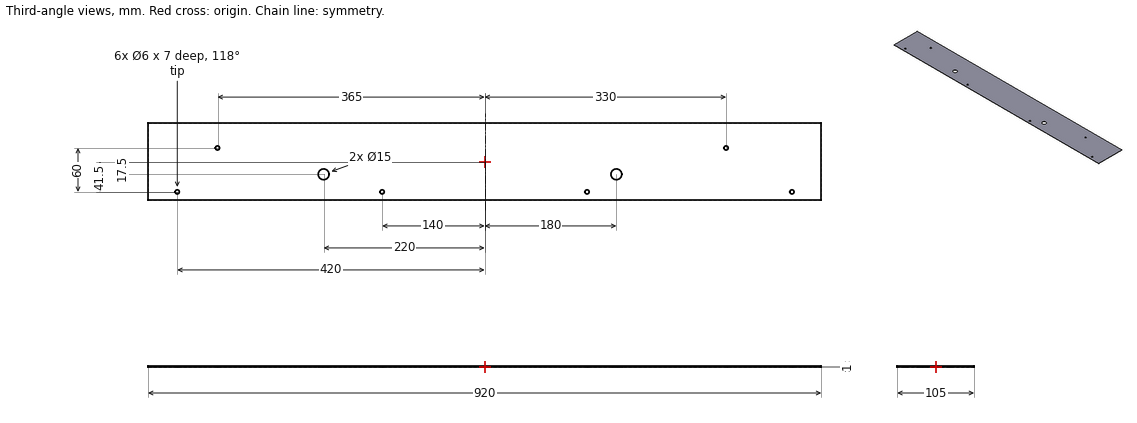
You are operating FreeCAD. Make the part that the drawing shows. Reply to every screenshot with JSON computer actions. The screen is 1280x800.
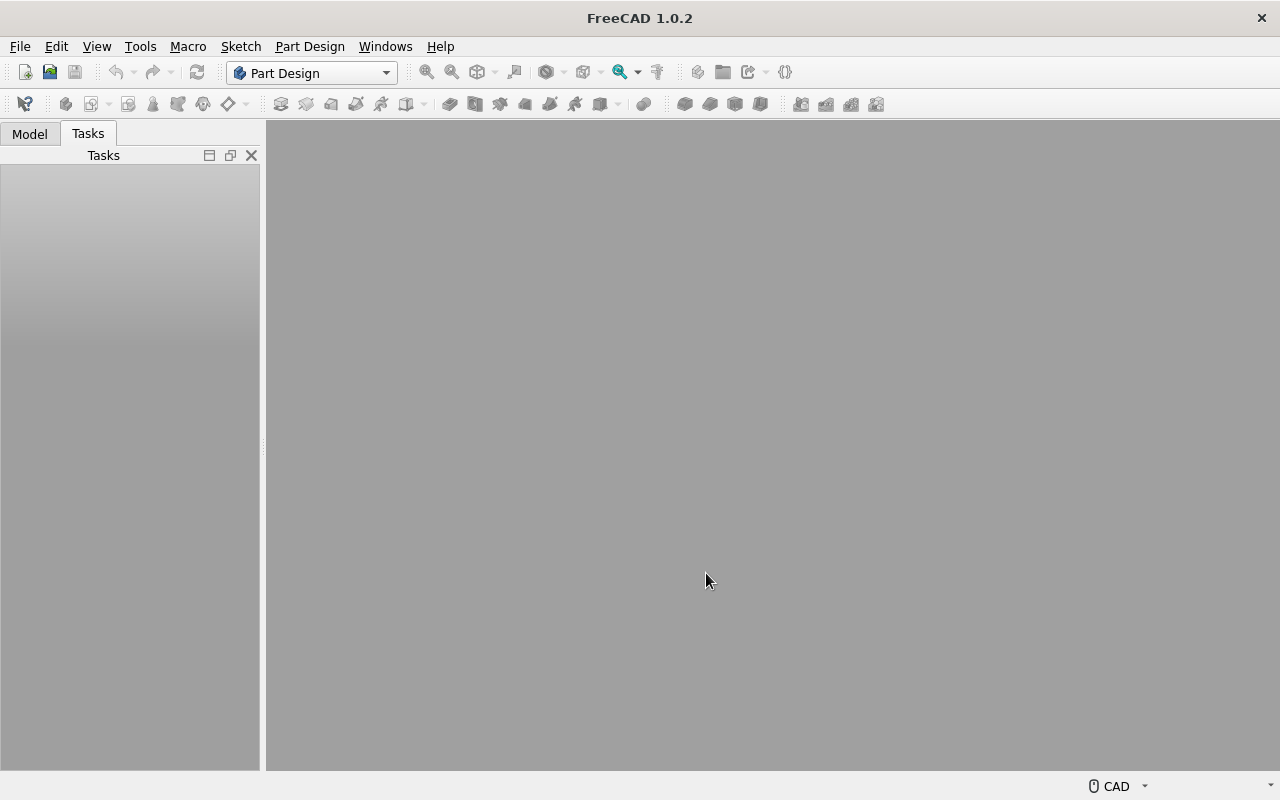
{"action": "left_click", "coordinate": [25, 72]}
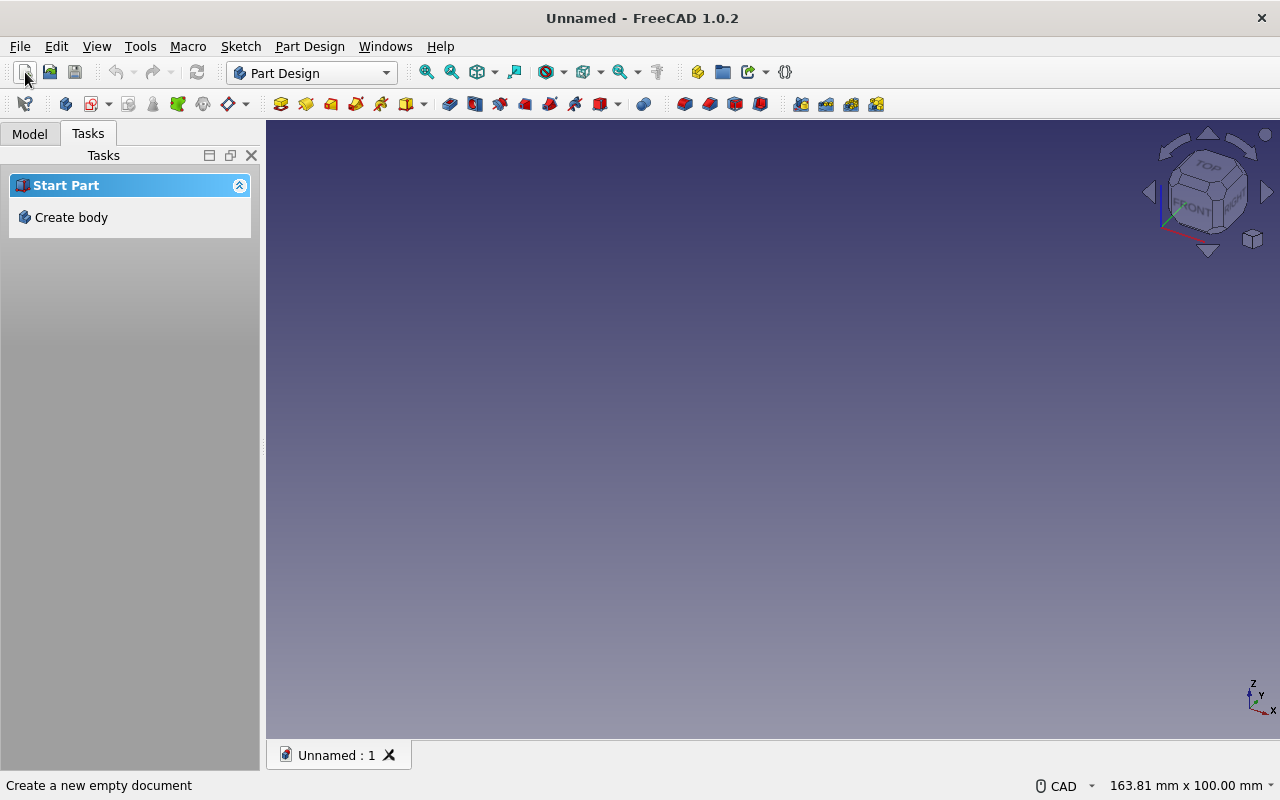
{"action": "left_click", "coordinate": [90, 104]}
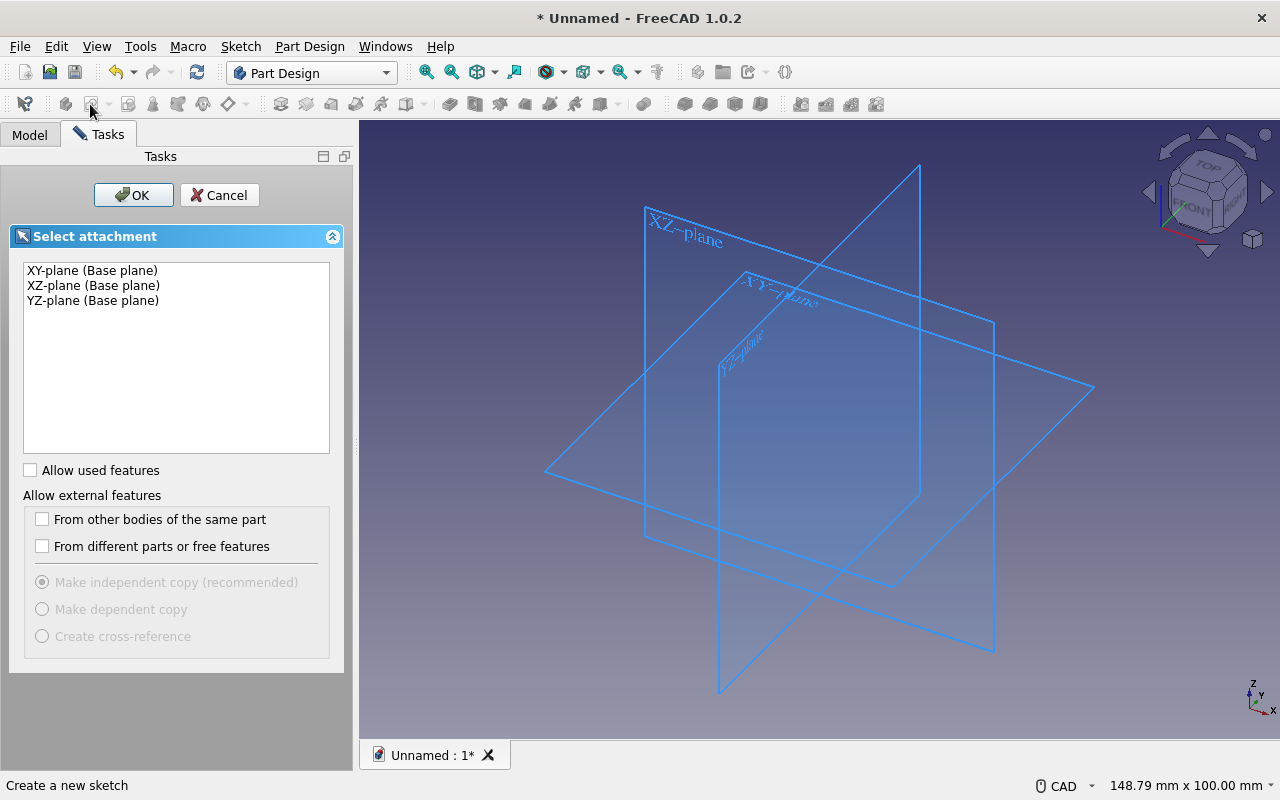
{"action": "left_click", "coordinate": [84, 286]}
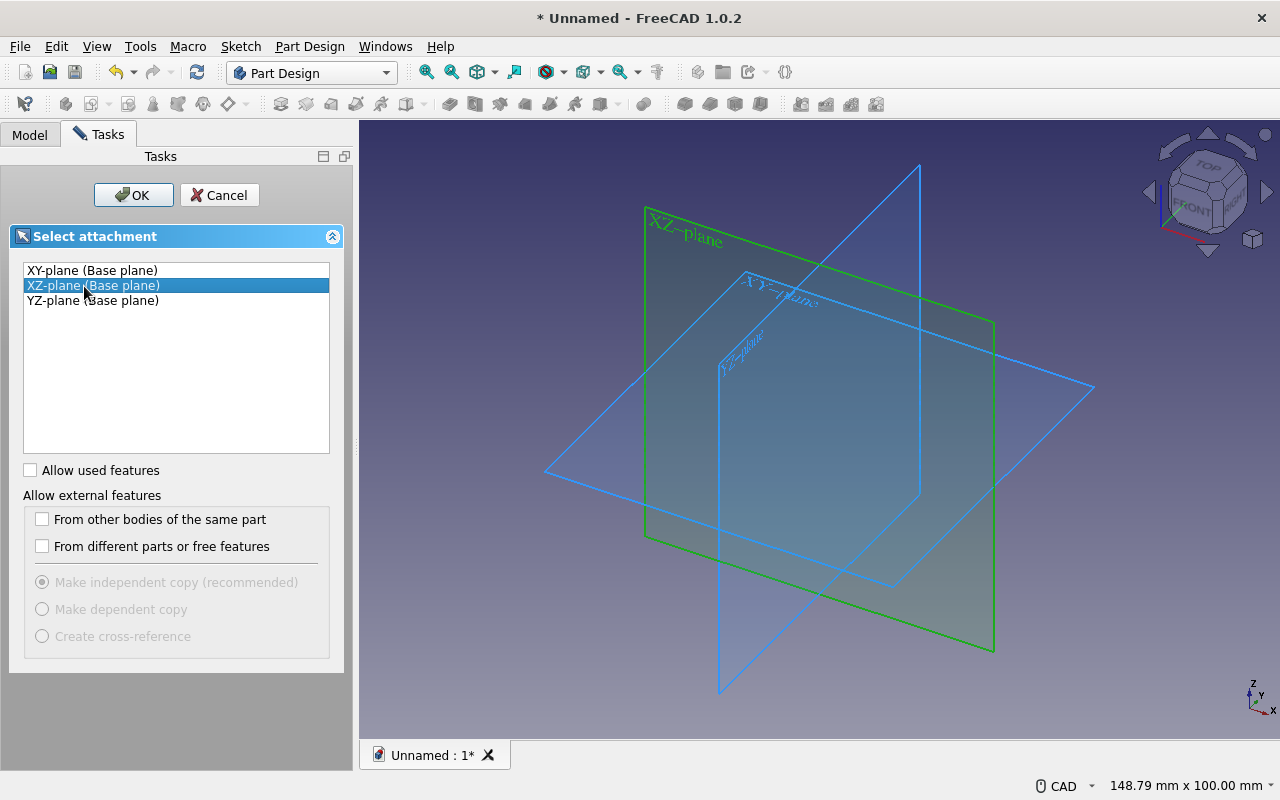
{"action": "left_click", "coordinate": [134, 195]}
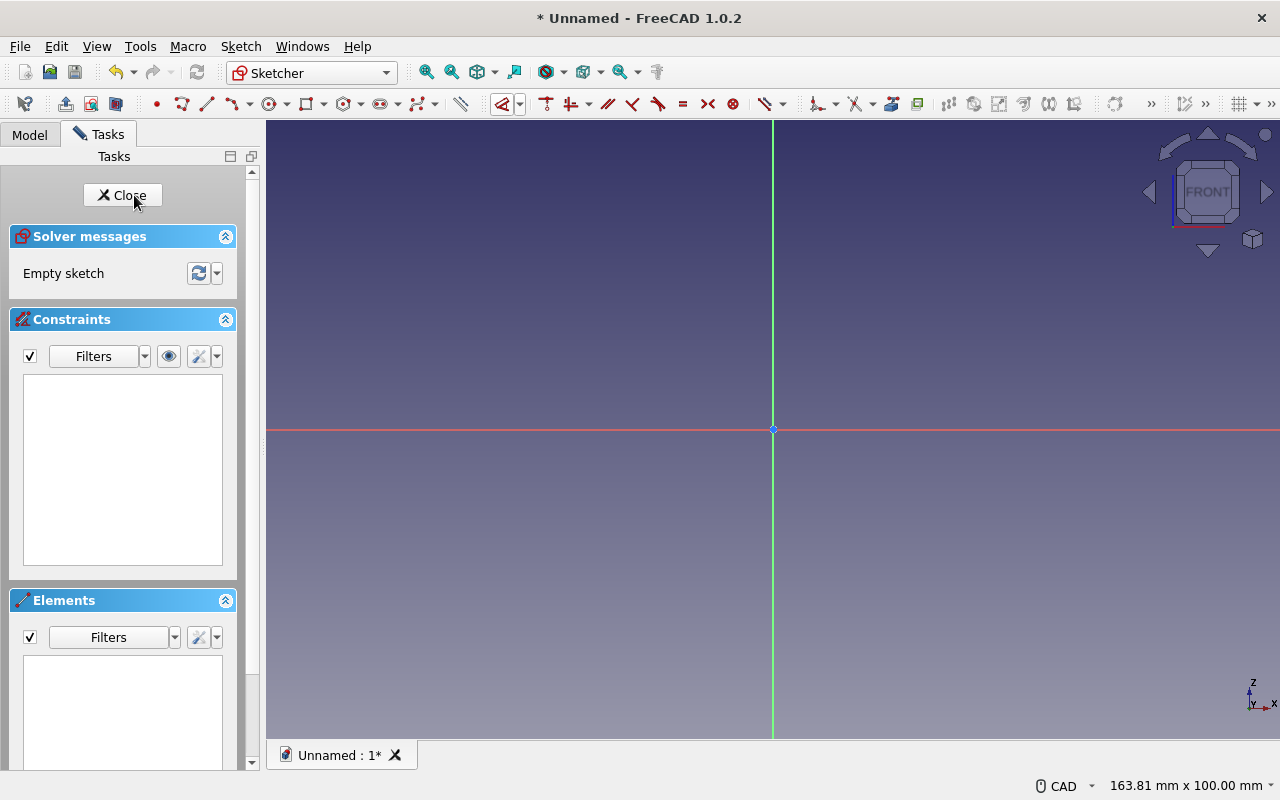
{"action": "scroll", "coordinate": [696, 430], "scroll_direction": "down", "scroll_amount": 11}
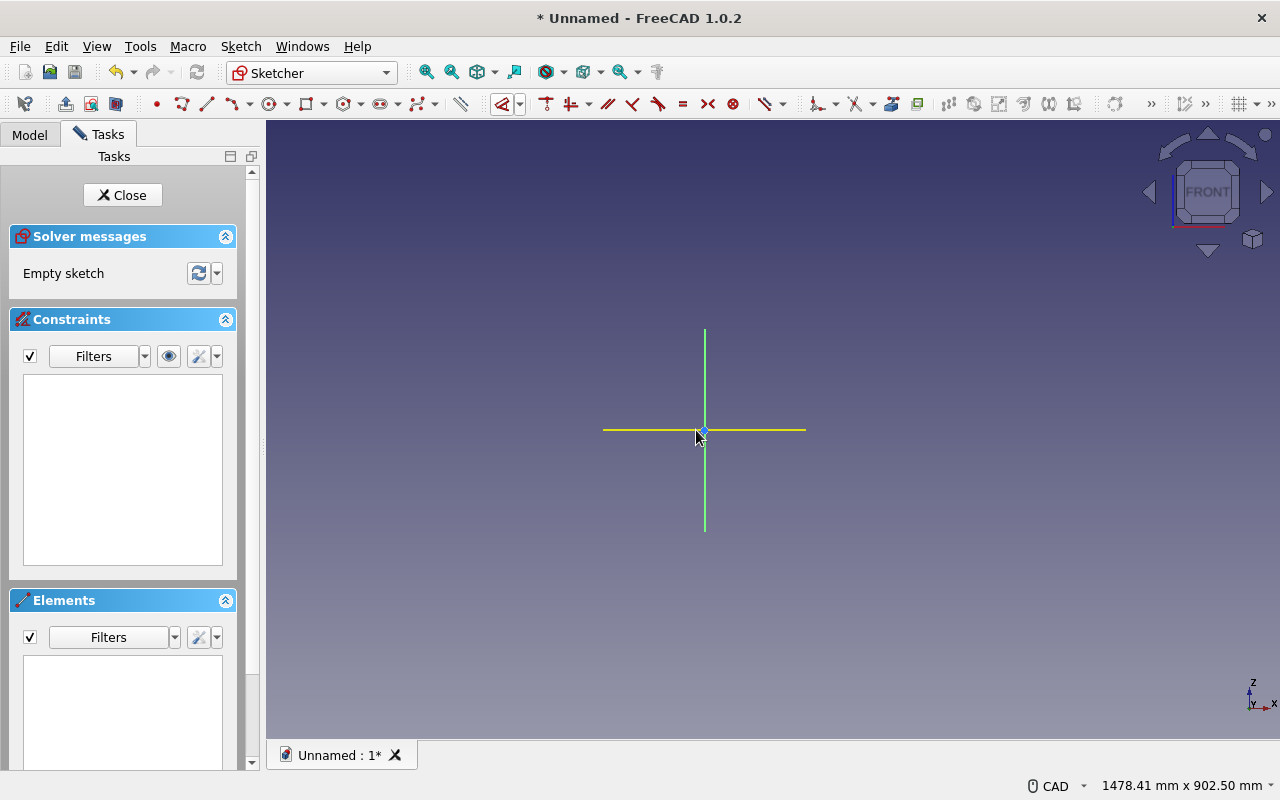
{"action": "key", "text": "g v"}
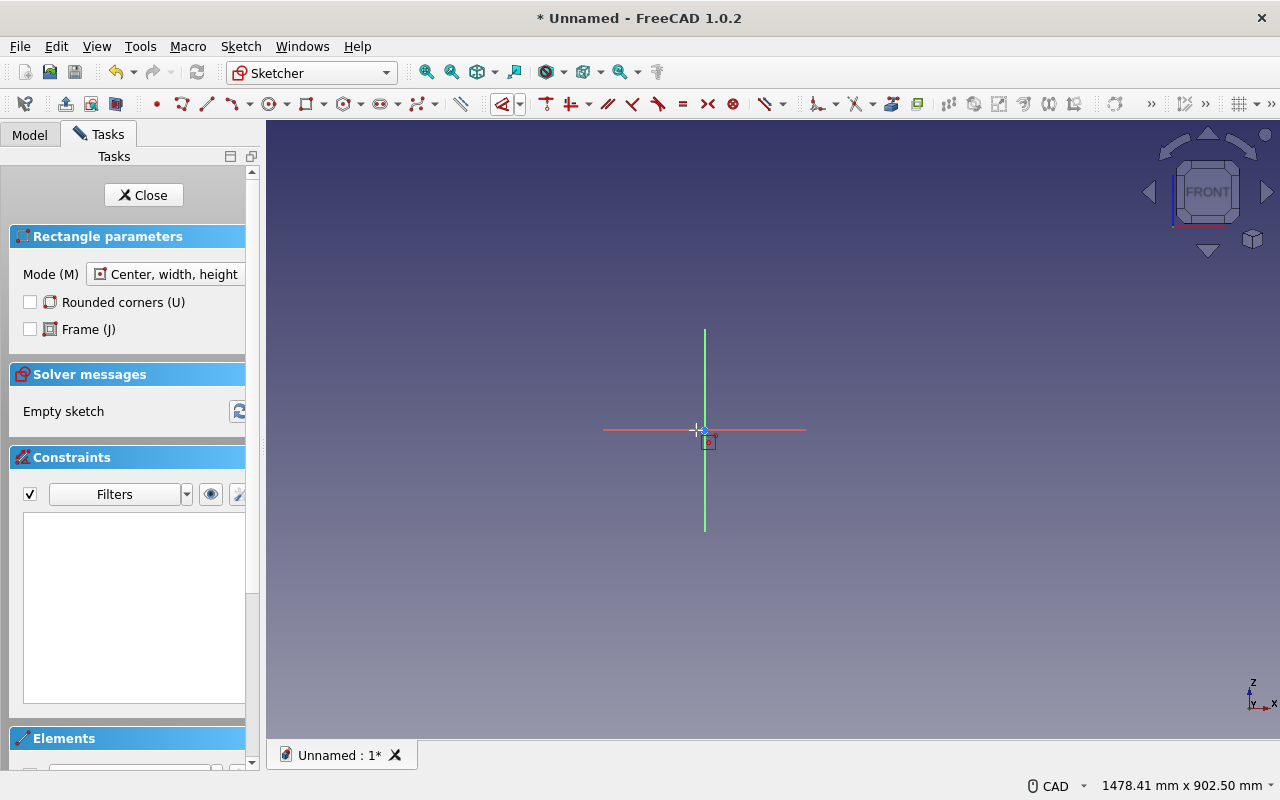
{"action": "scroll", "coordinate": [705, 430], "scroll_direction": "up", "scroll_amount": 20}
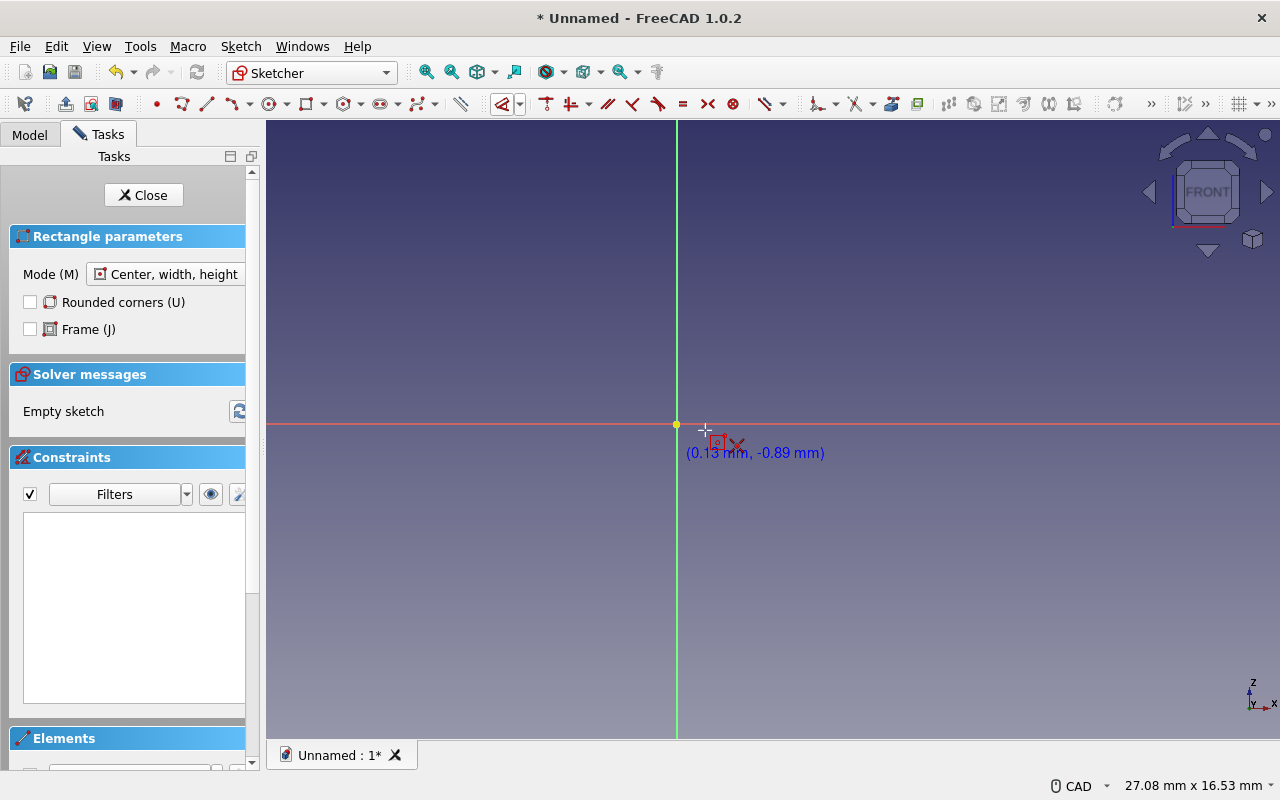
{"action": "scroll", "coordinate": [704, 430], "scroll_direction": "down", "scroll_amount": 15}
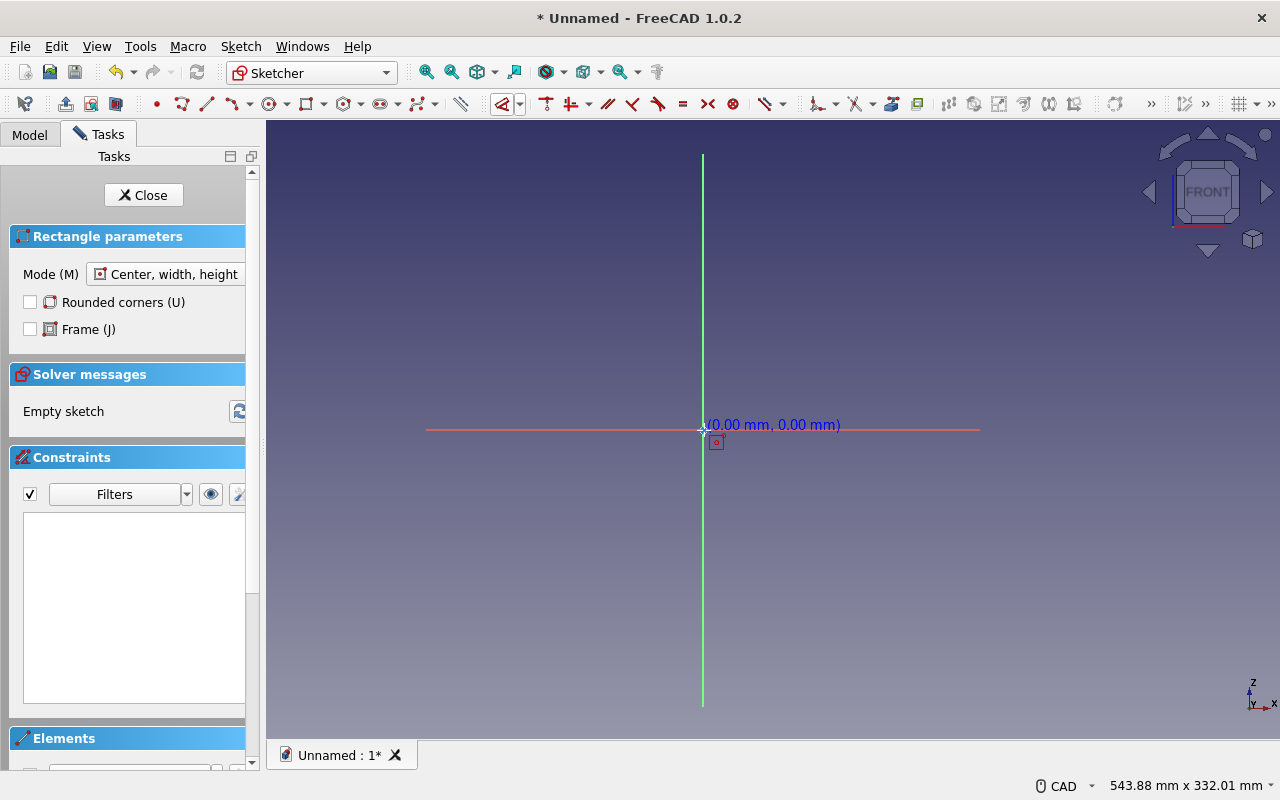
{"action": "scroll", "coordinate": [705, 429], "scroll_direction": "down", "scroll_amount": 5}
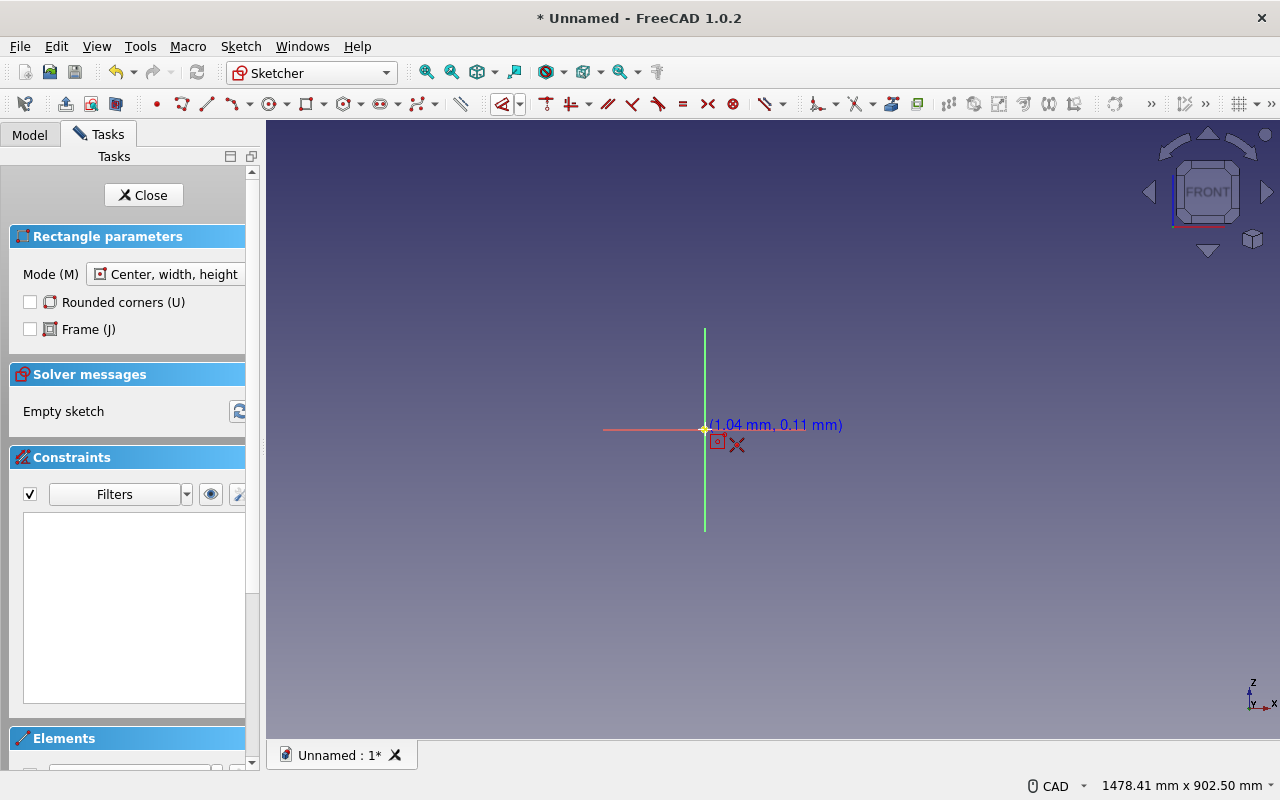
{"action": "left_click", "coordinate": [705, 430]}